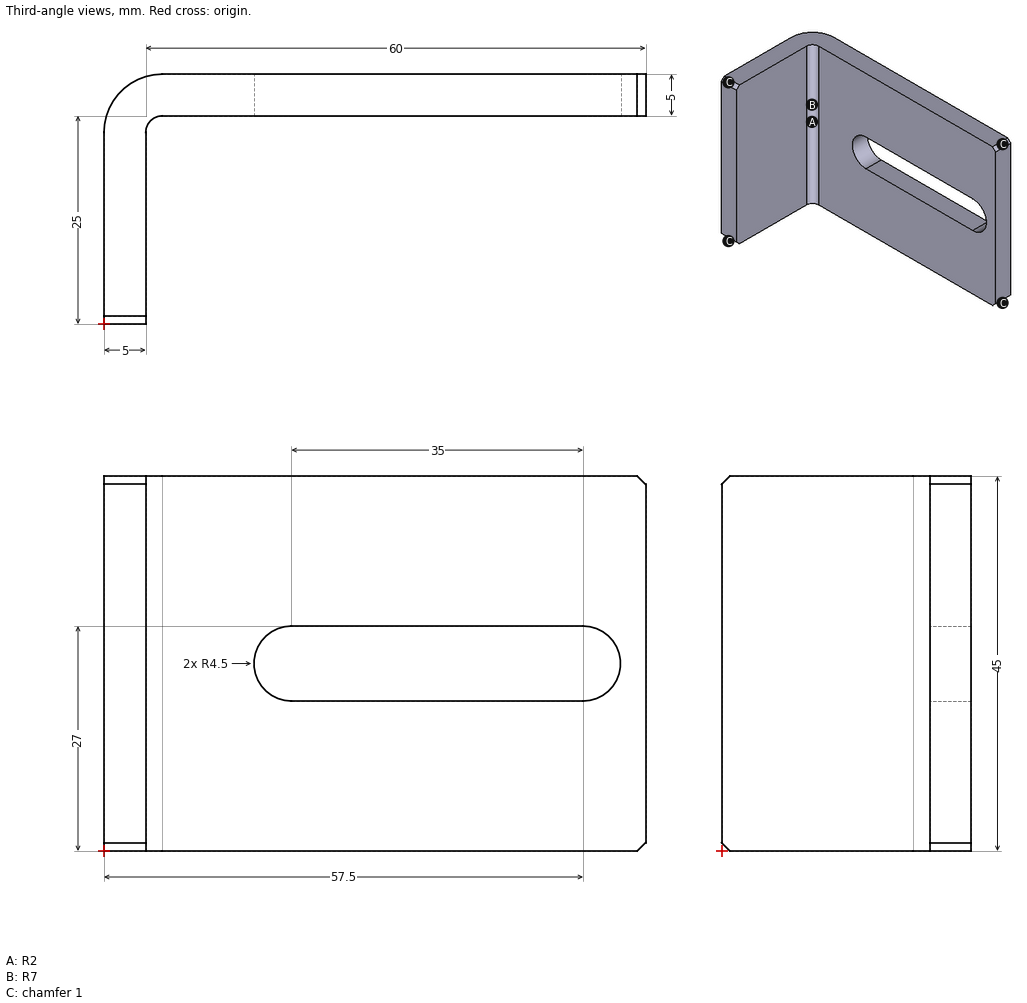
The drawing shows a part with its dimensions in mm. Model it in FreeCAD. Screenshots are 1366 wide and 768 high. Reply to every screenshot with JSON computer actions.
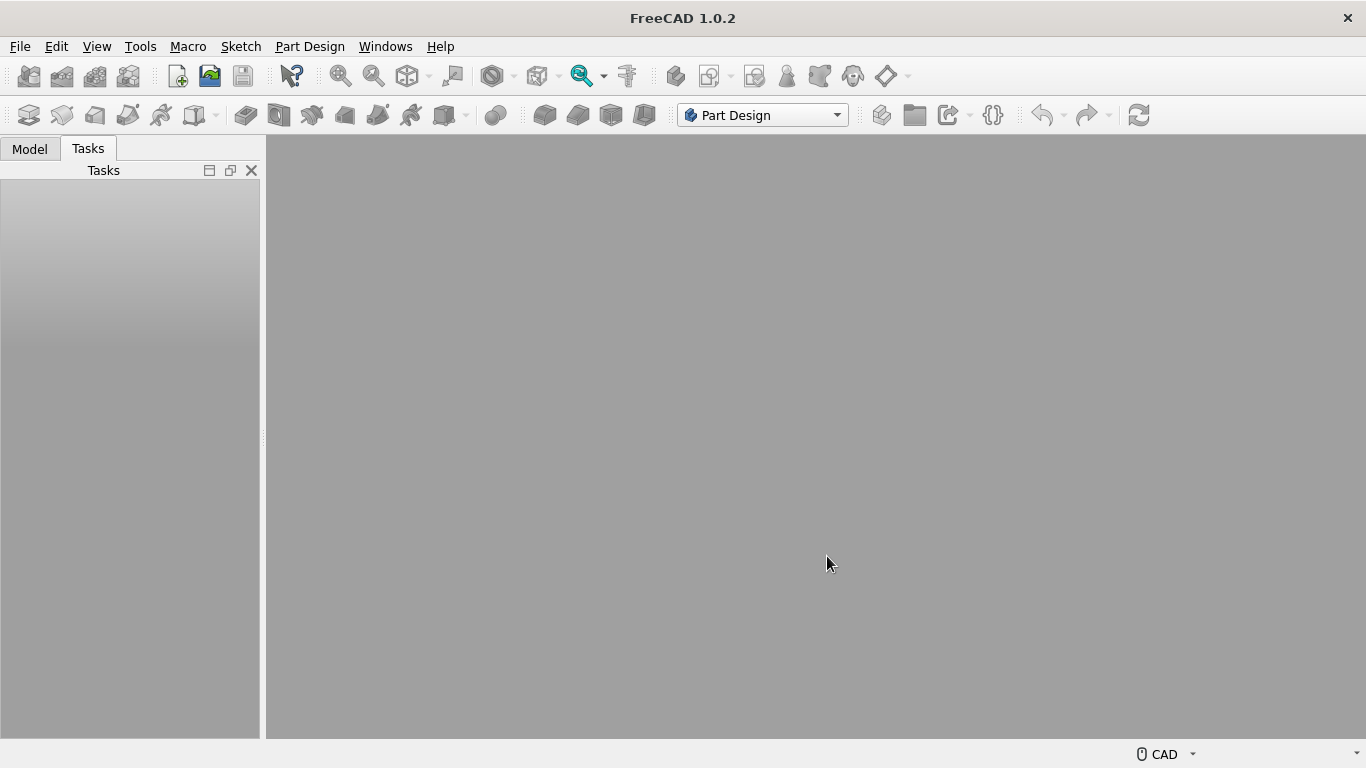
{"action": "left_click", "coordinate": [177, 76]}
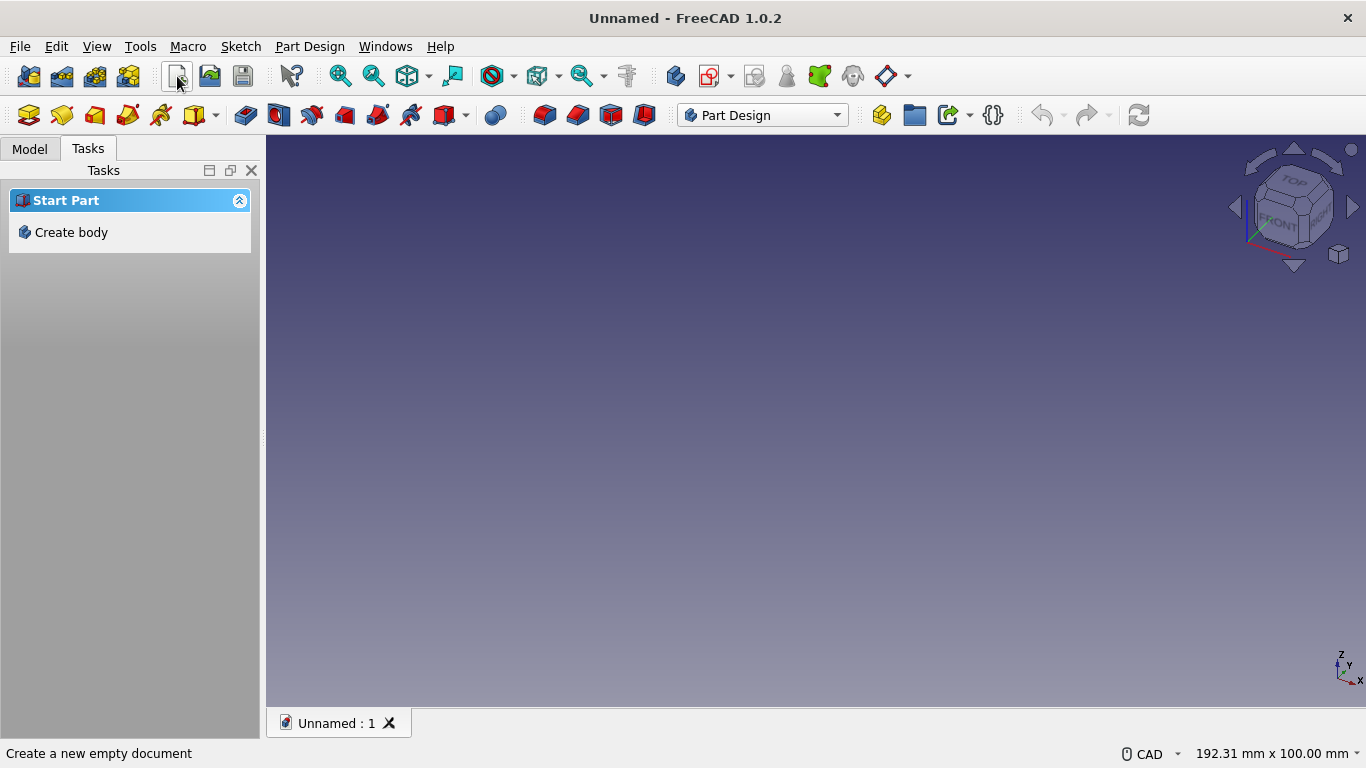
{"action": "left_click", "coordinate": [708, 76]}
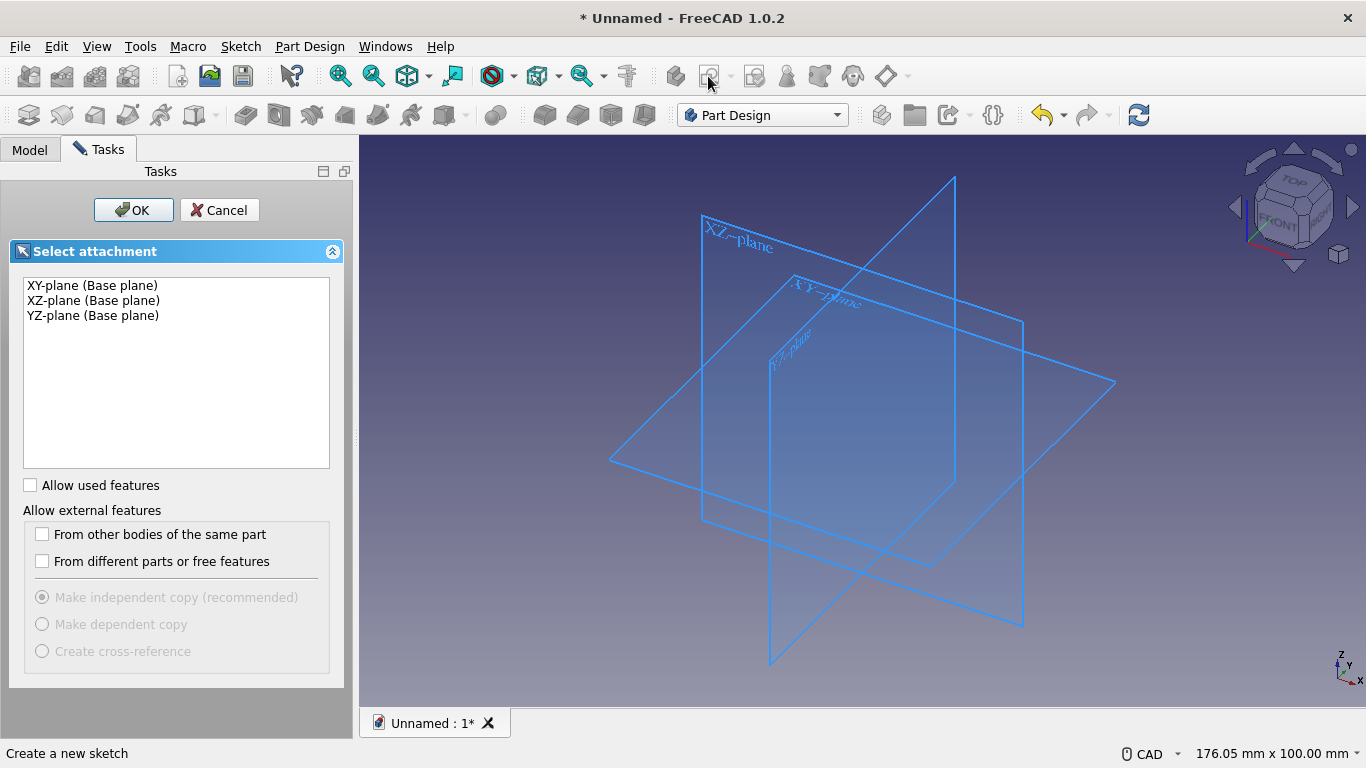
{"action": "left_click", "coordinate": [84, 286]}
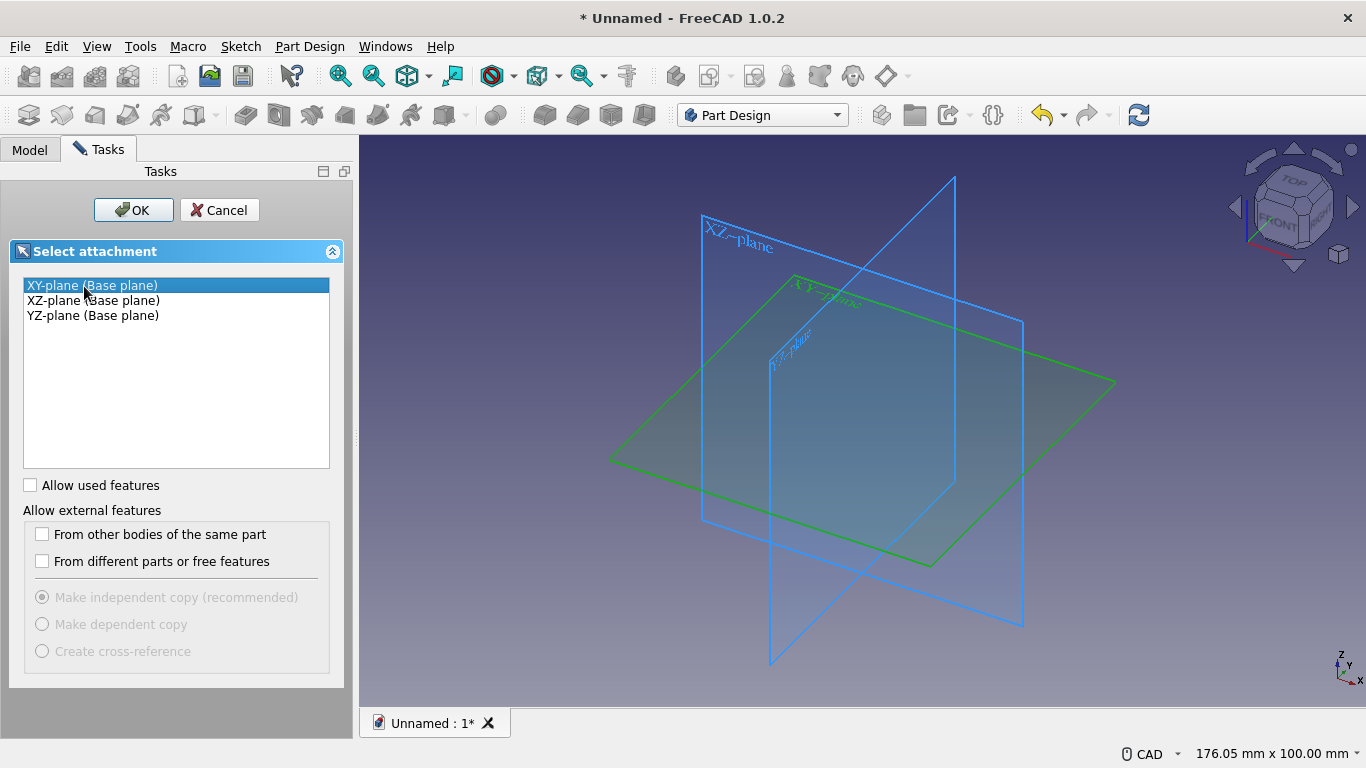
{"action": "left_click", "coordinate": [134, 210]}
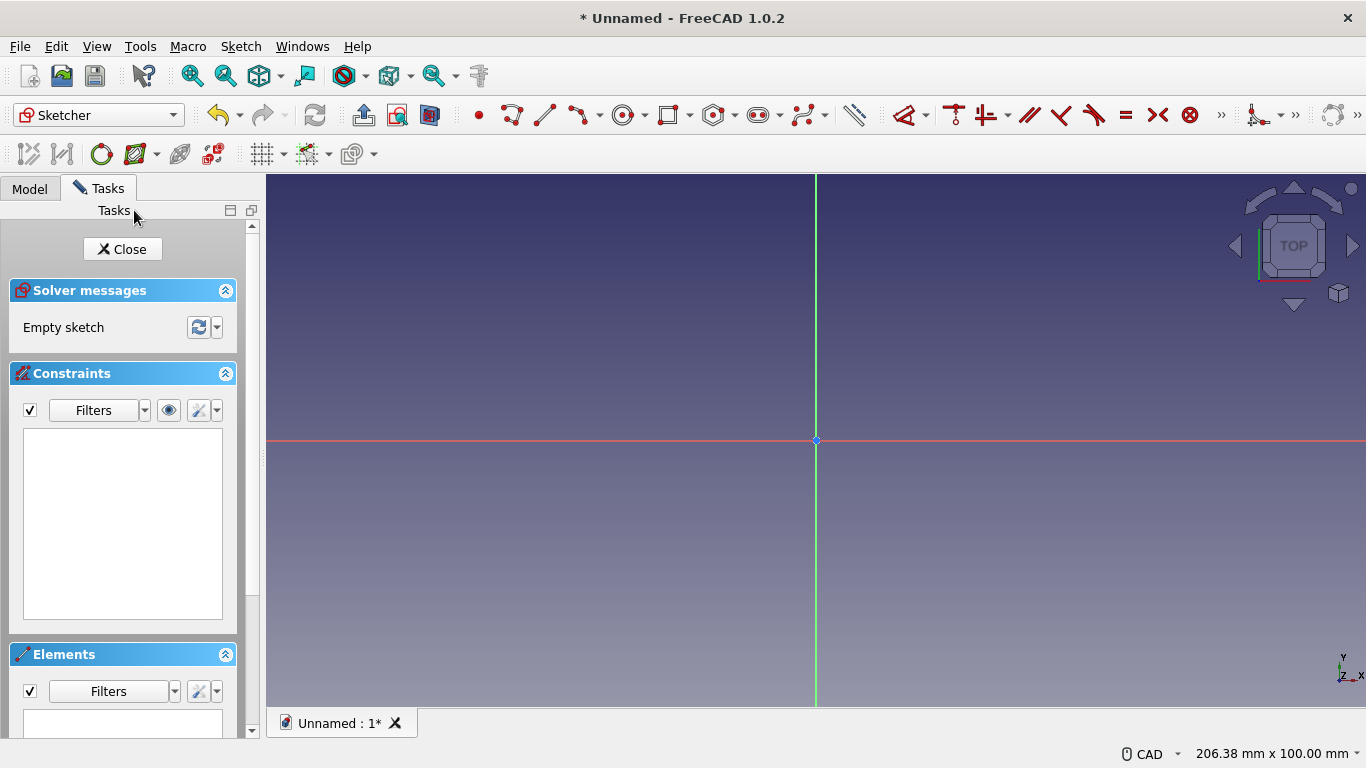
{"action": "scroll", "coordinate": [1201, 263], "scroll_direction": "up", "scroll_amount": 3}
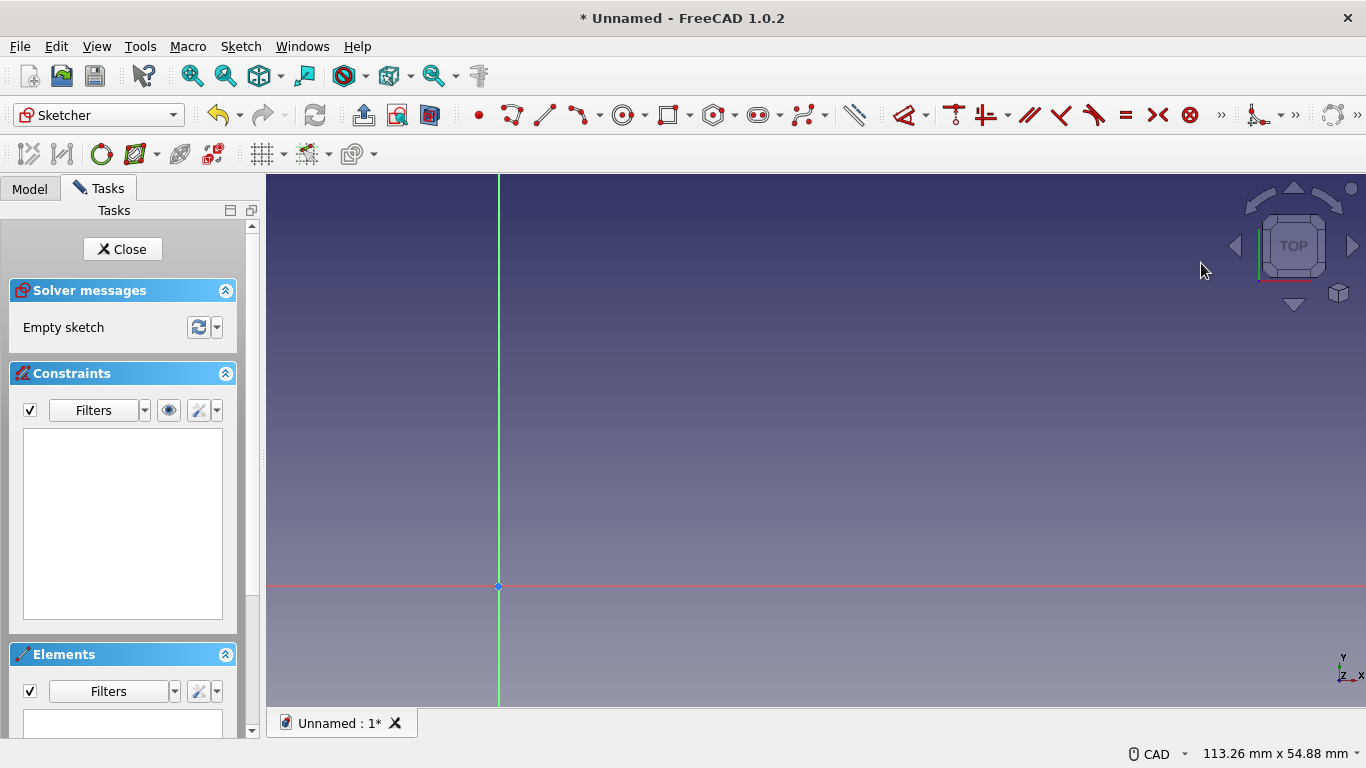
{"action": "left_click", "coordinate": [512, 116]}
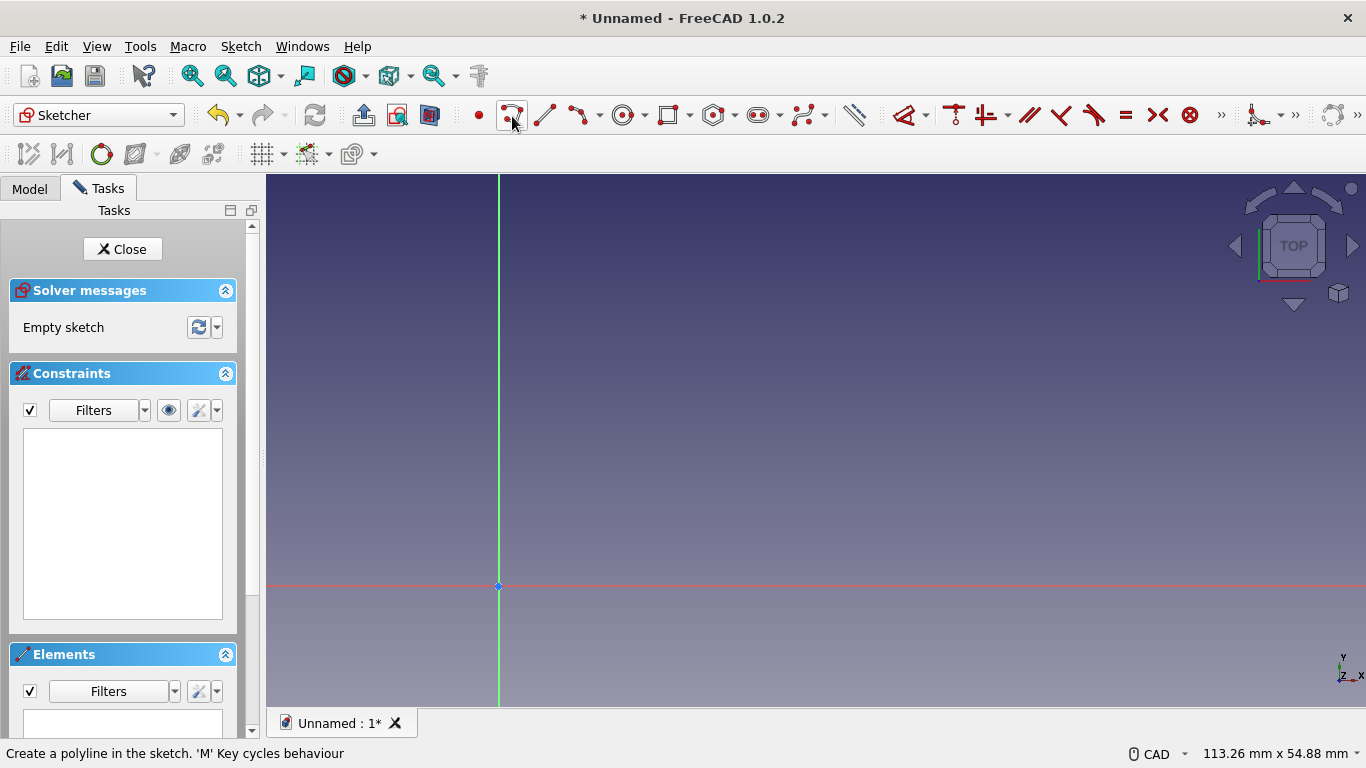
{"action": "left_click", "coordinate": [499, 586]}
{"action": "left_click", "coordinate": [547, 577]}
{"action": "left_click", "coordinate": [547, 343]}
{"action": "left_click", "coordinate": [1130, 343]}
{"action": "left_click", "coordinate": [1130, 295]}
{"action": "left_click", "coordinate": [508, 295]}
{"action": "left_click", "coordinate": [499, 586]}
{"action": "key", "text": "Escape"}
{"action": "key", "text": "Escape"}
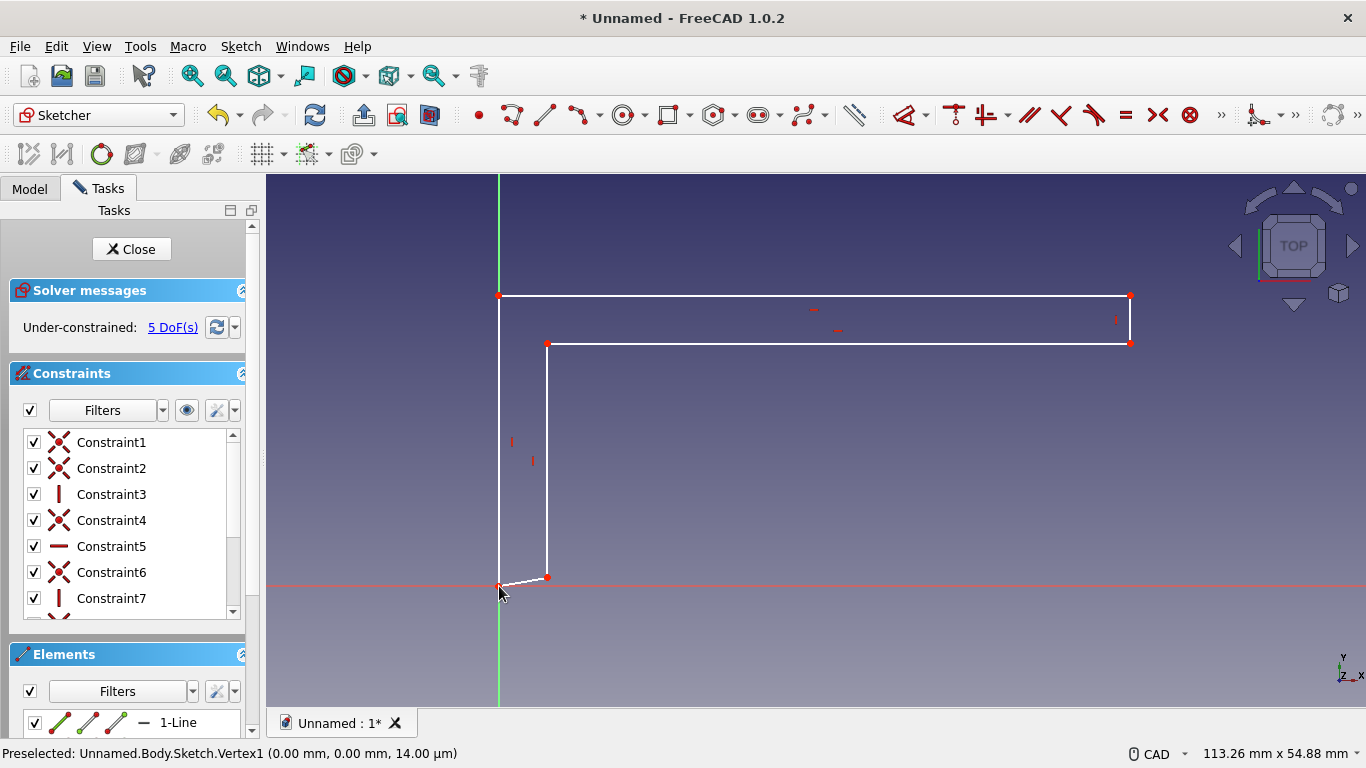
{"action": "left_click", "coordinate": [513, 584]}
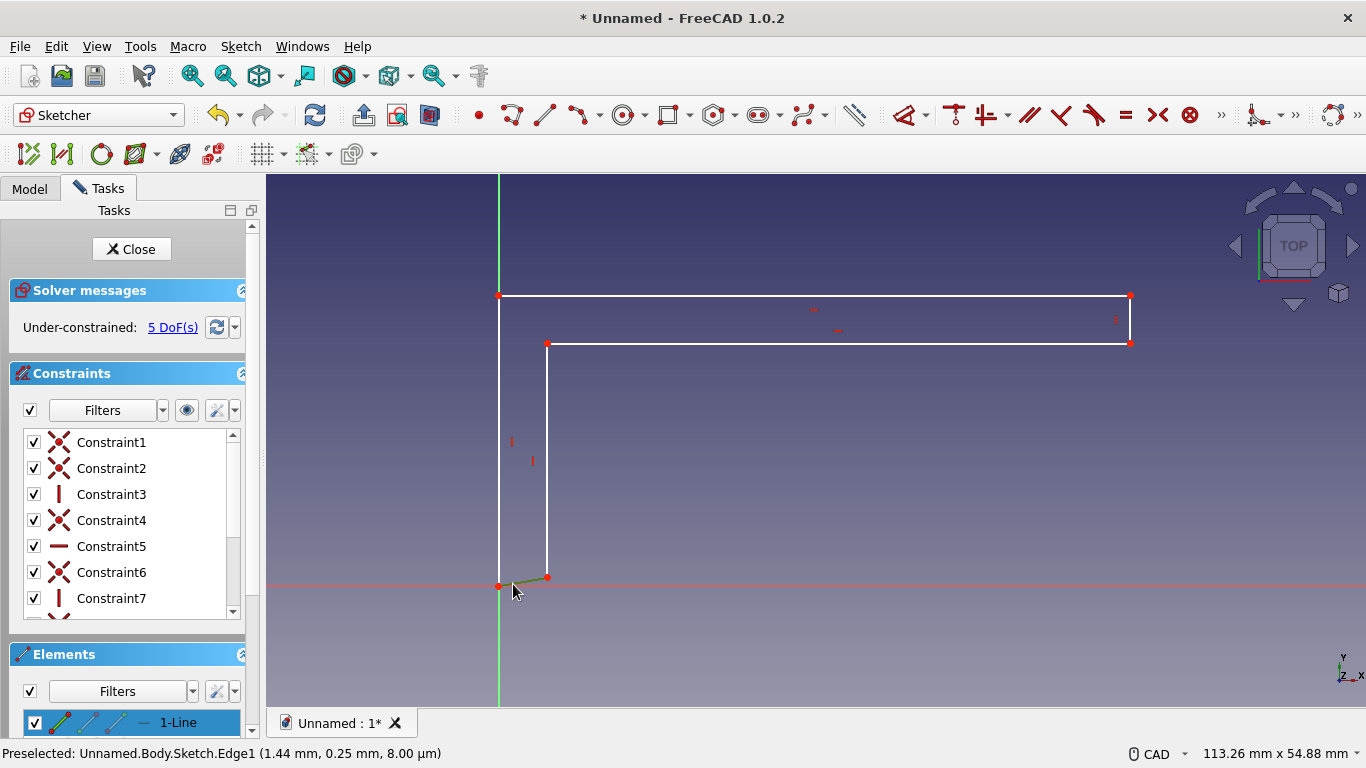
{"action": "left_click", "coordinate": [1008, 116]}